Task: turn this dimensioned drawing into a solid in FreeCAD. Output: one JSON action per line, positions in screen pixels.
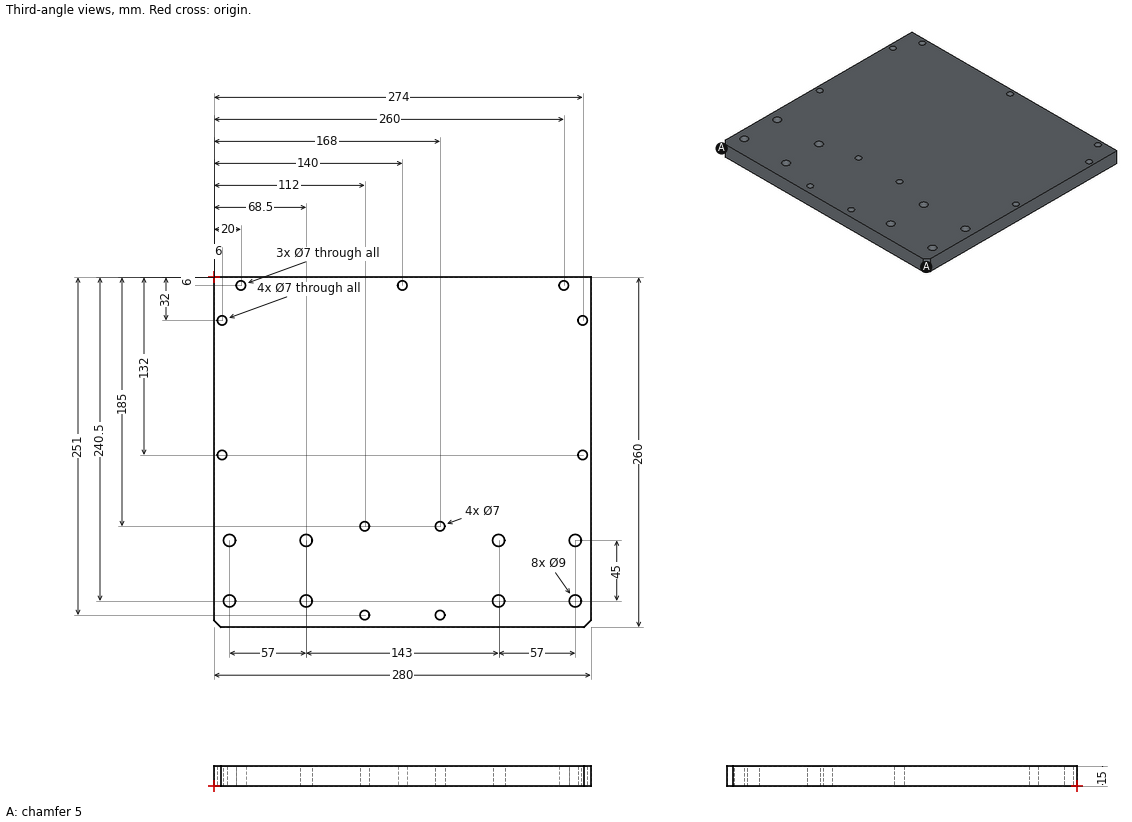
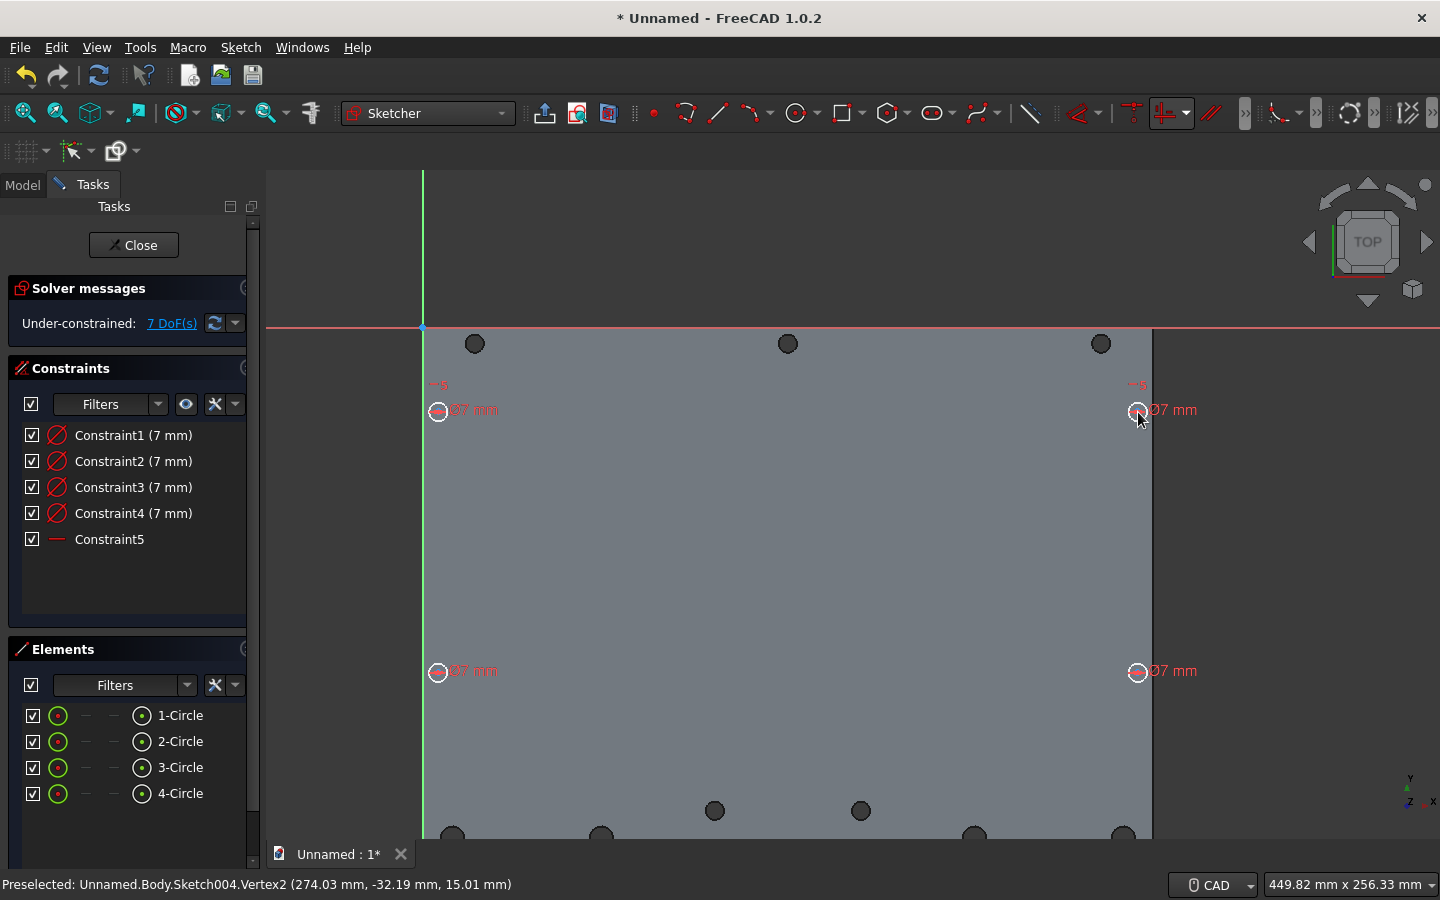
{"action": "left_click", "coordinate": [1138, 412]}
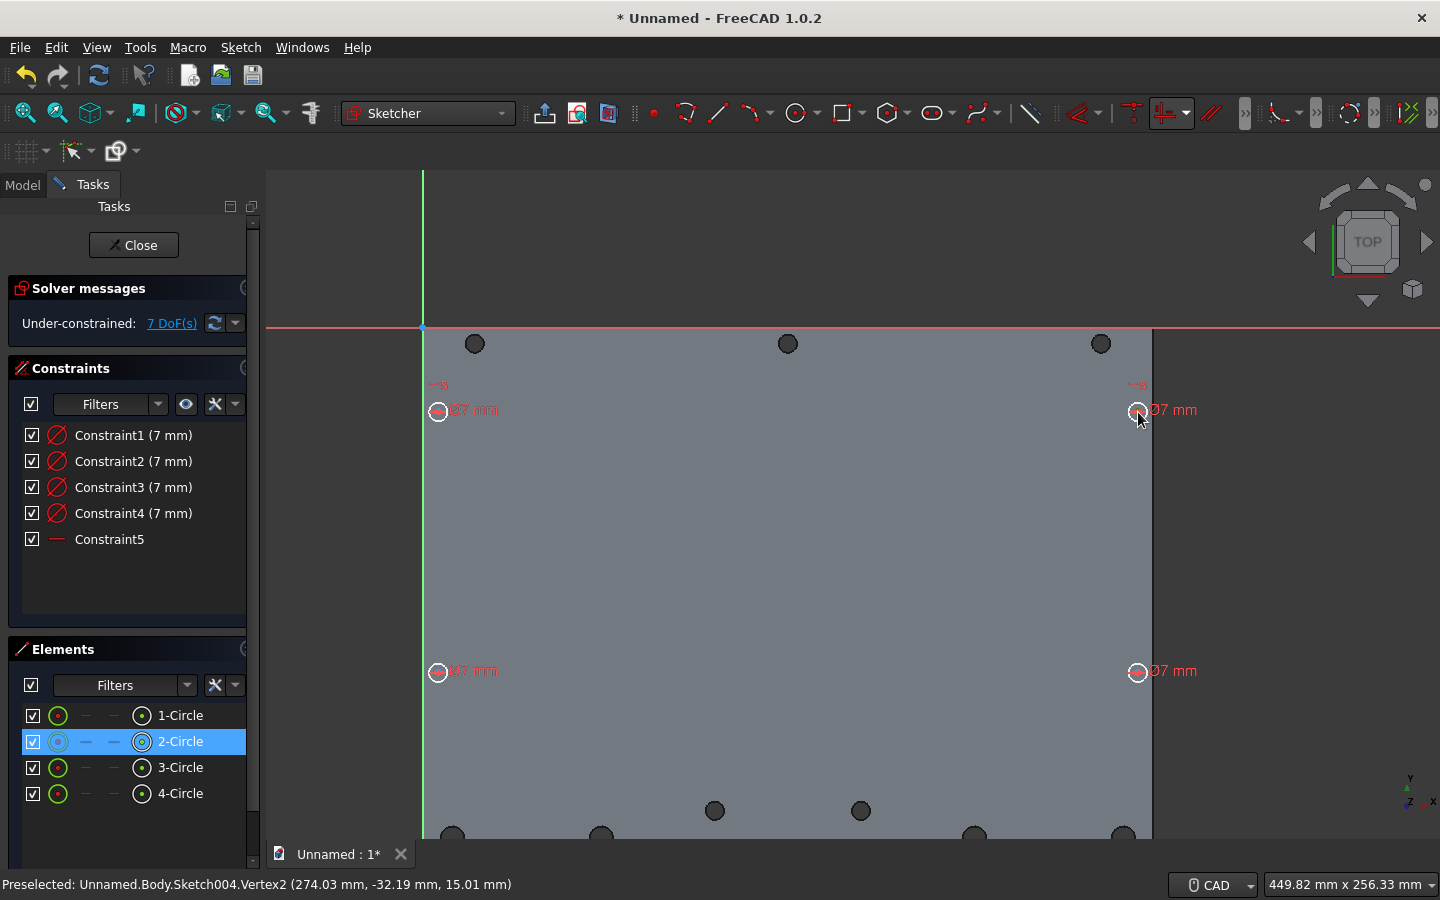
{"action": "left_click", "coordinate": [1138, 673]}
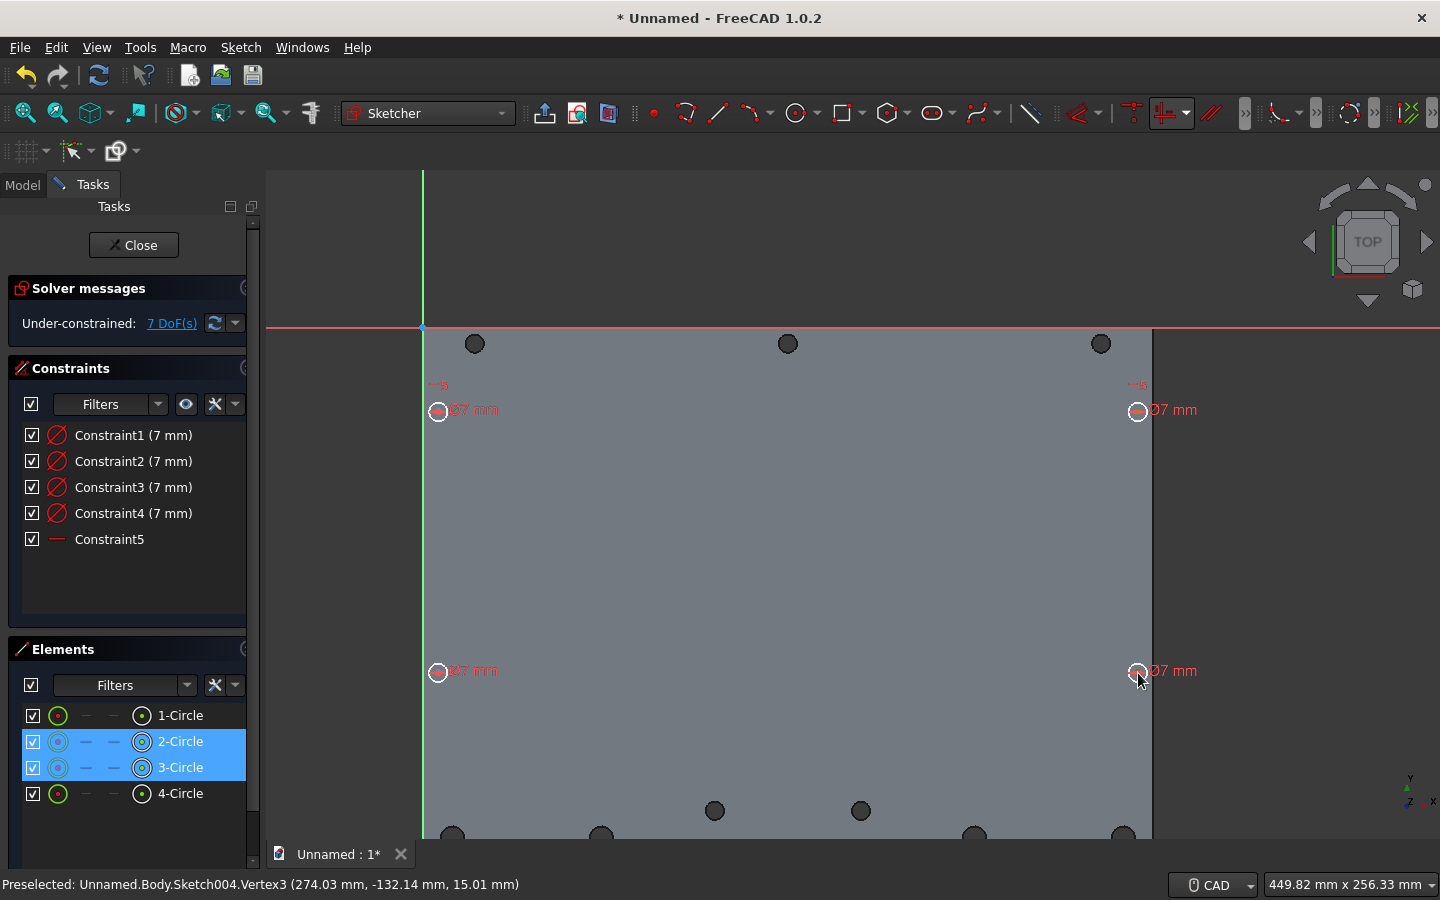
{"action": "left_click", "coordinate": [1188, 114]}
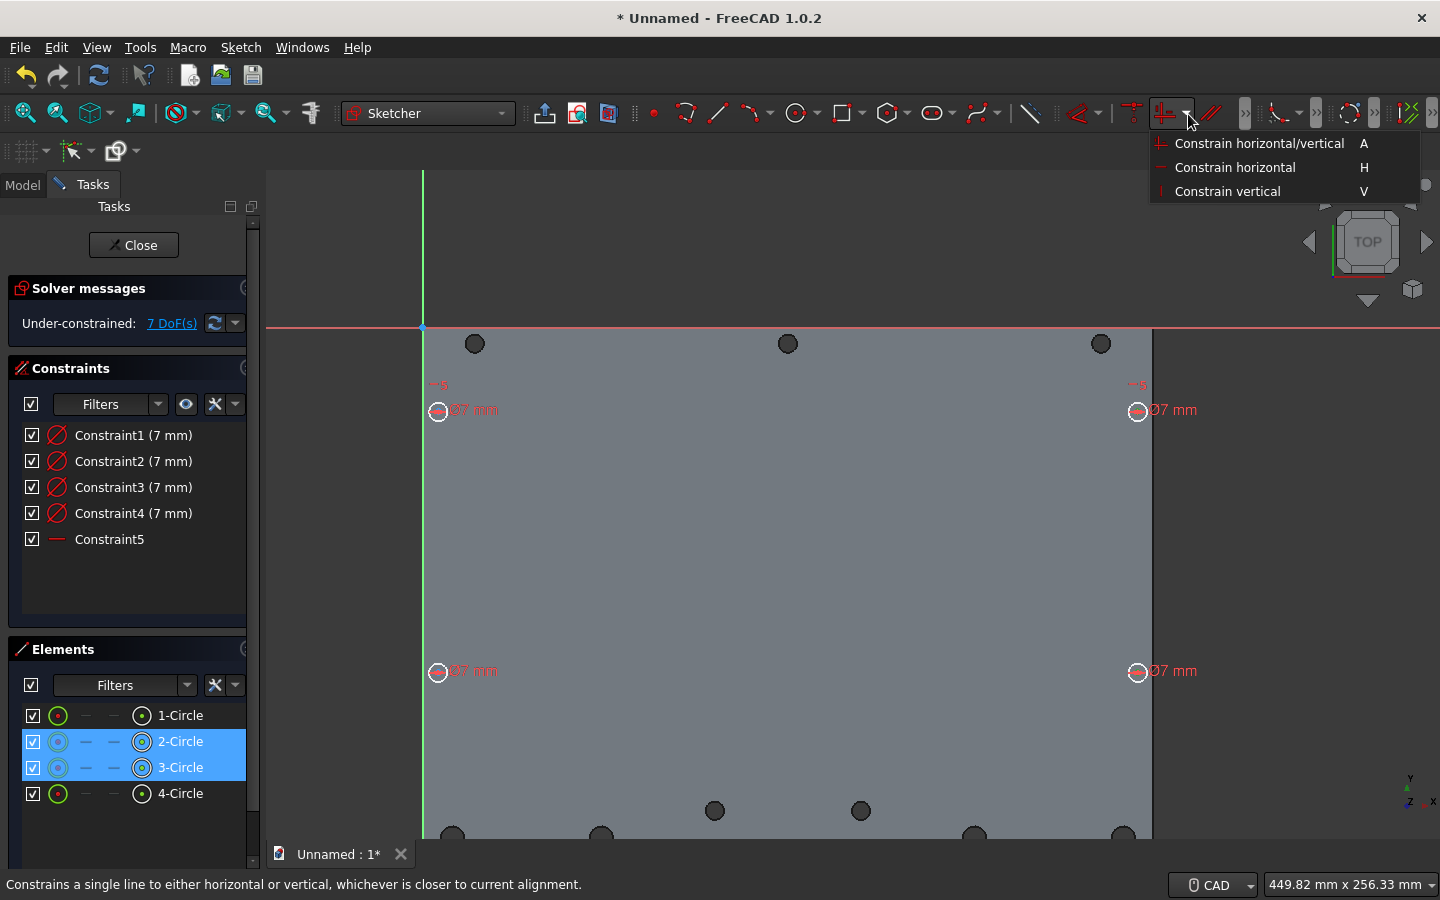
{"action": "left_click", "coordinate": [1285, 191]}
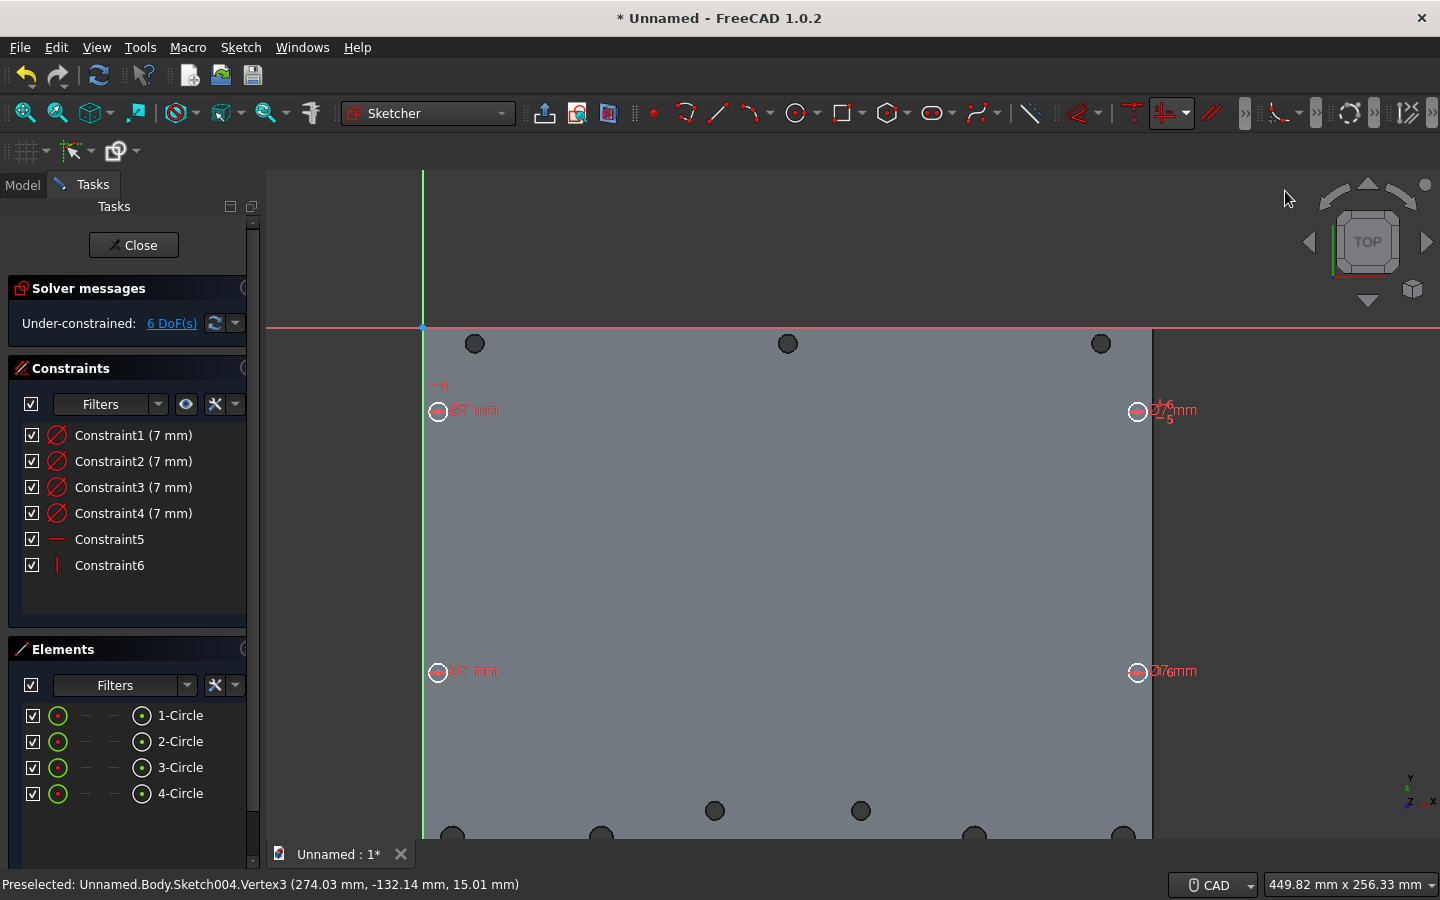
{"action": "left_click", "coordinate": [438, 412]}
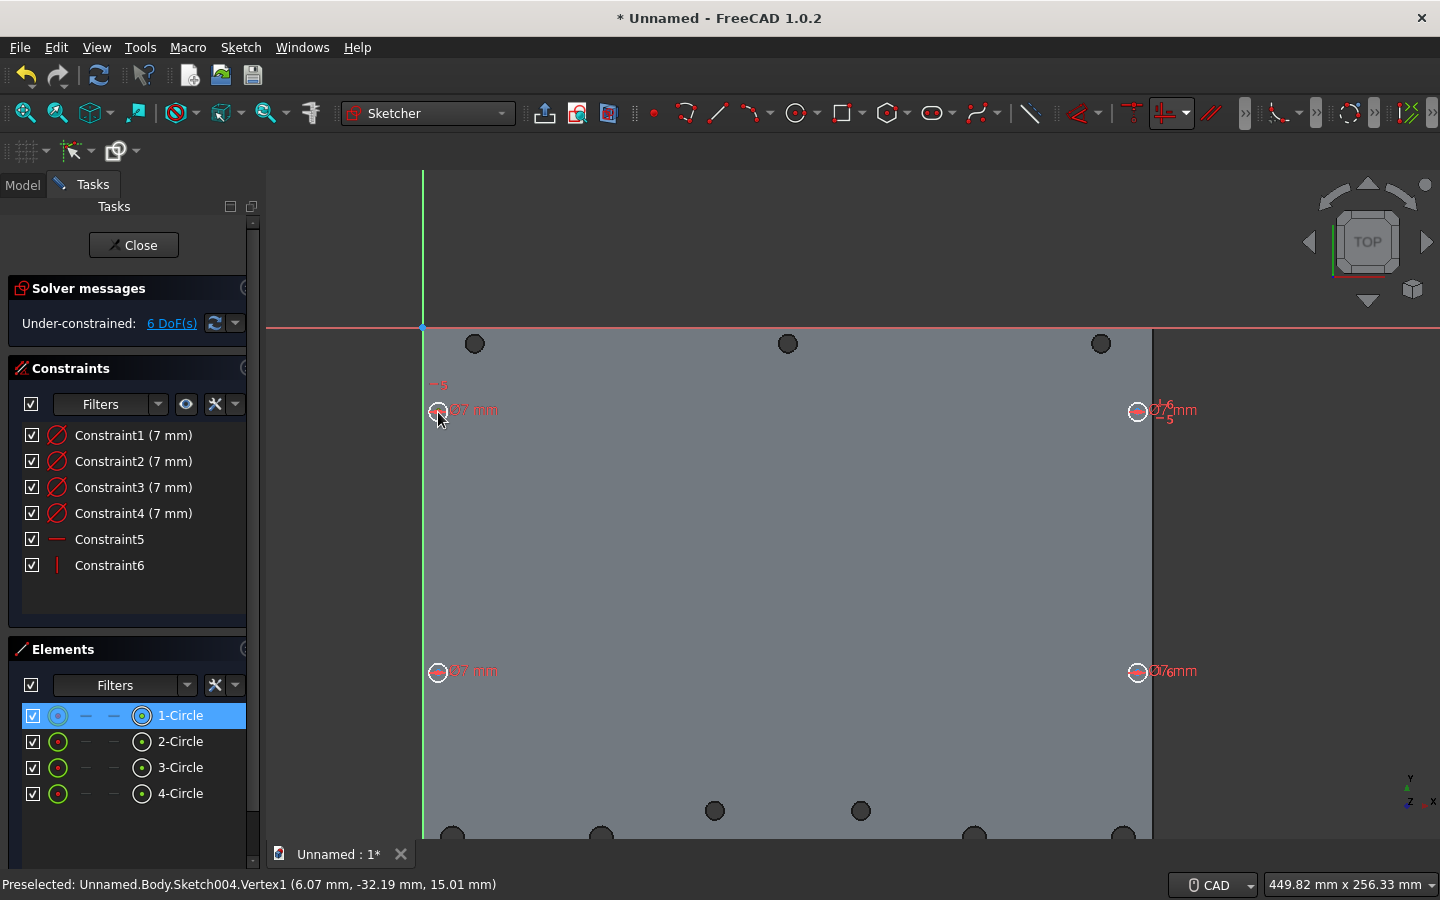
{"action": "left_click", "coordinate": [438, 673]}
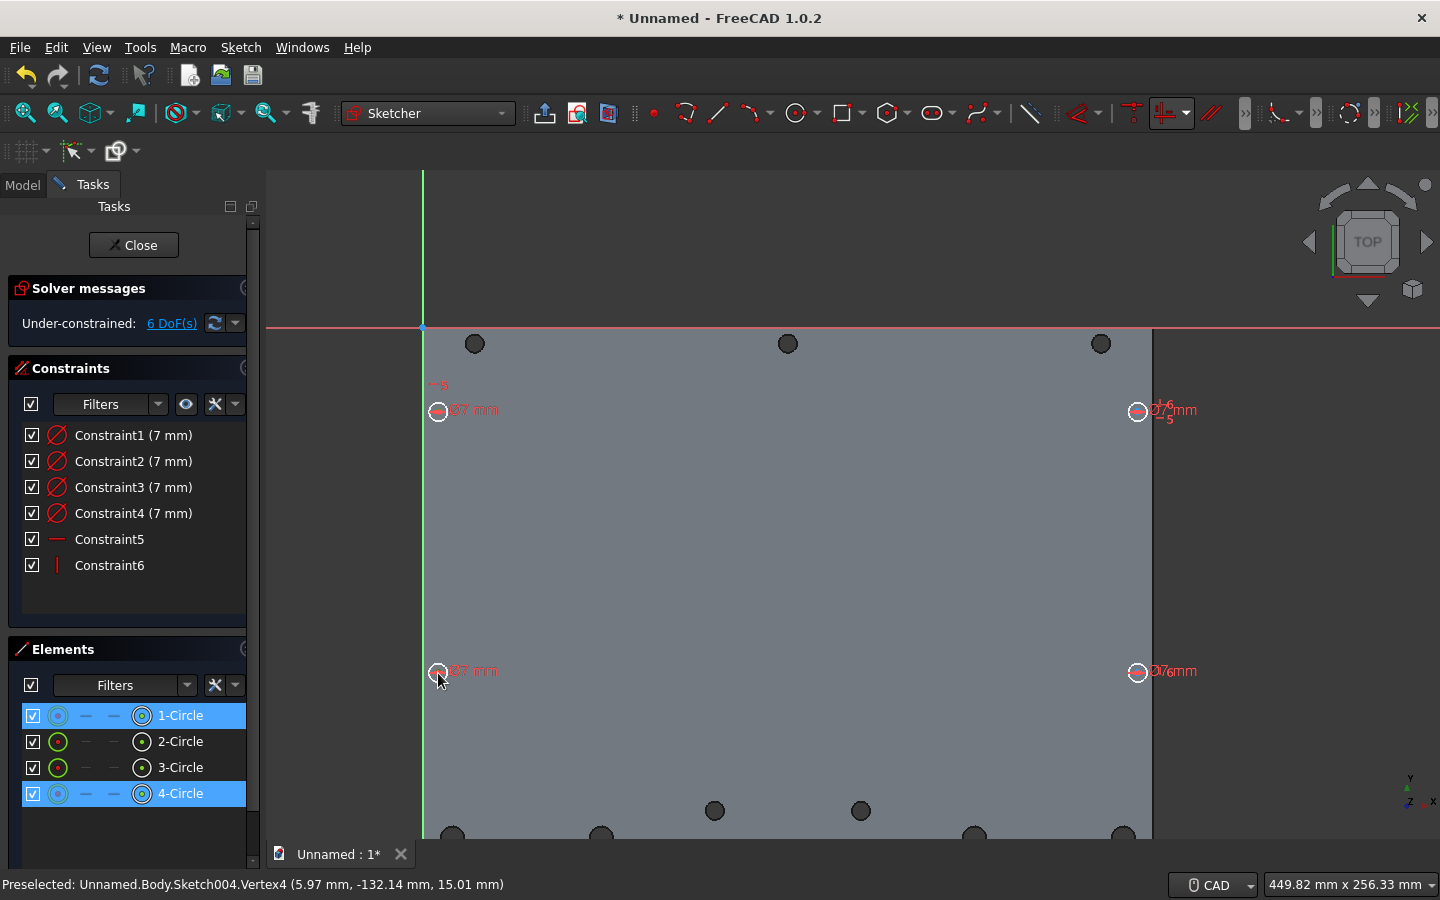
{"action": "key", "text": "v"}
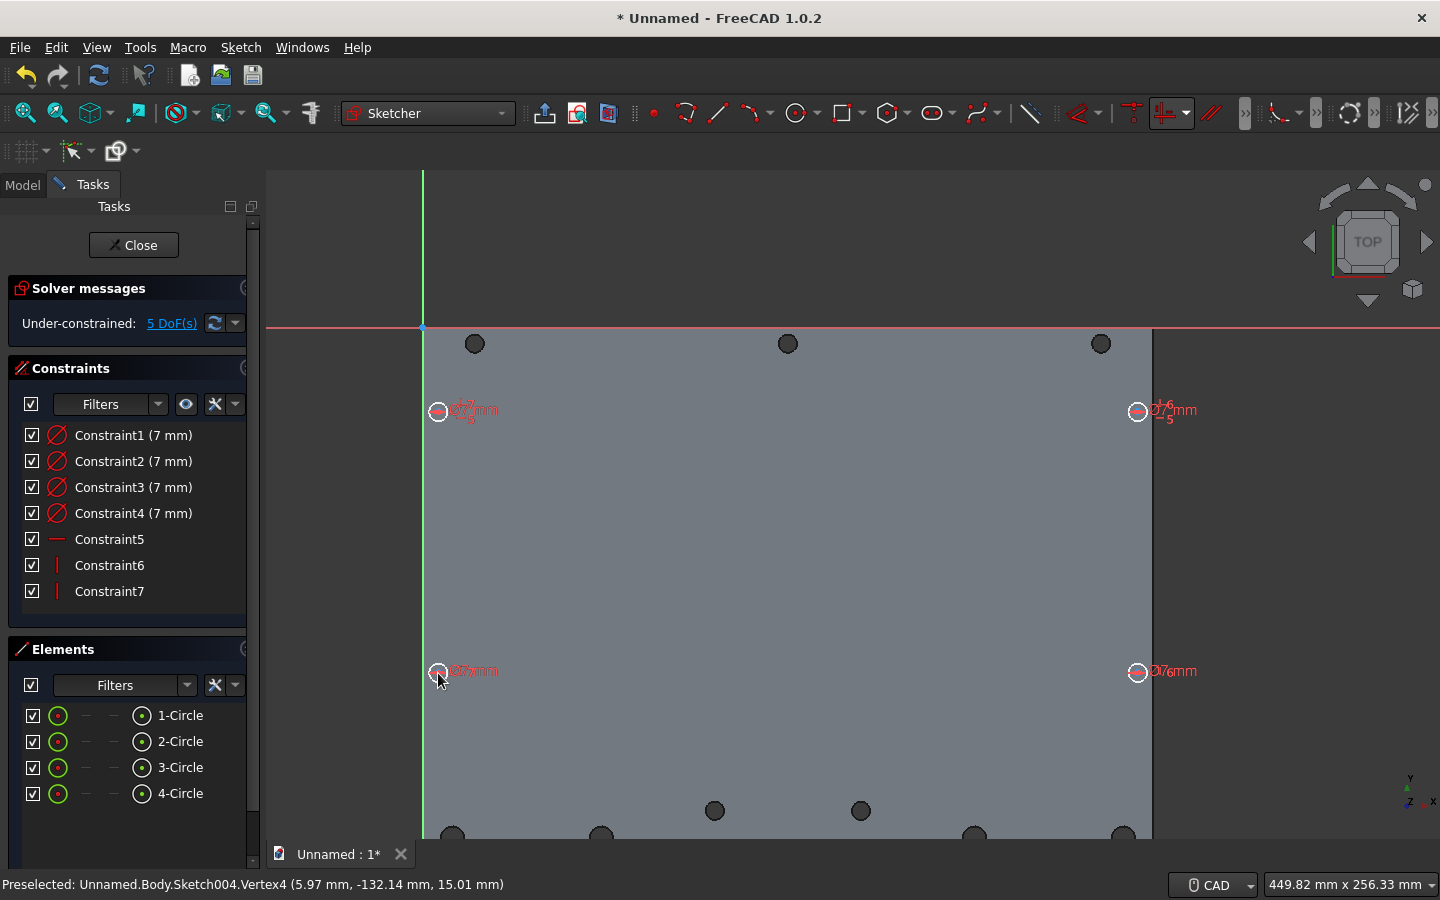
{"action": "left_click", "coordinate": [1138, 673]}